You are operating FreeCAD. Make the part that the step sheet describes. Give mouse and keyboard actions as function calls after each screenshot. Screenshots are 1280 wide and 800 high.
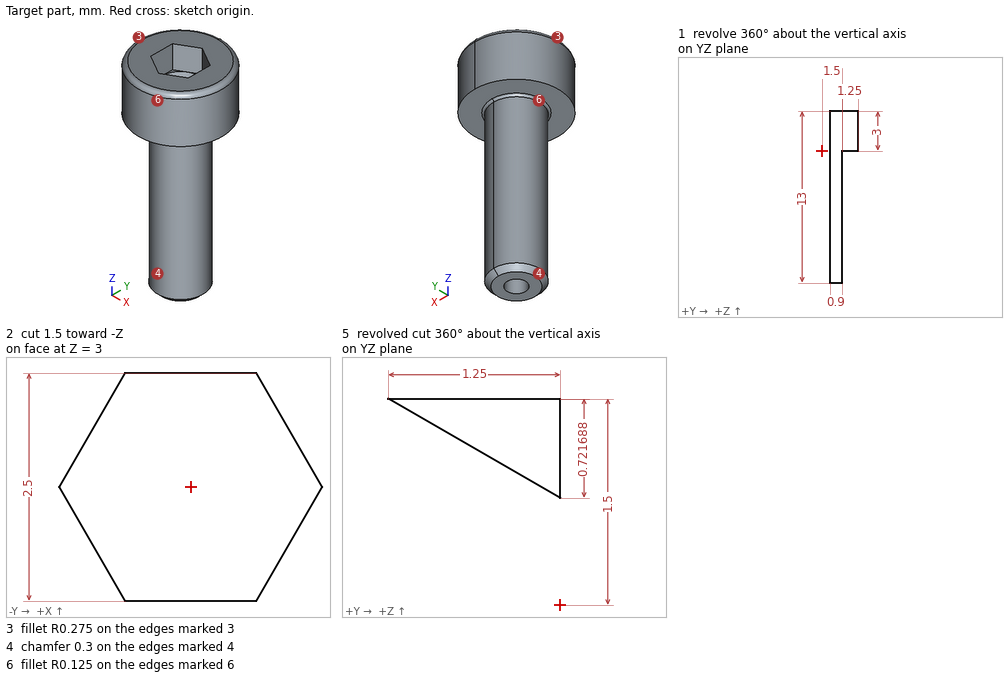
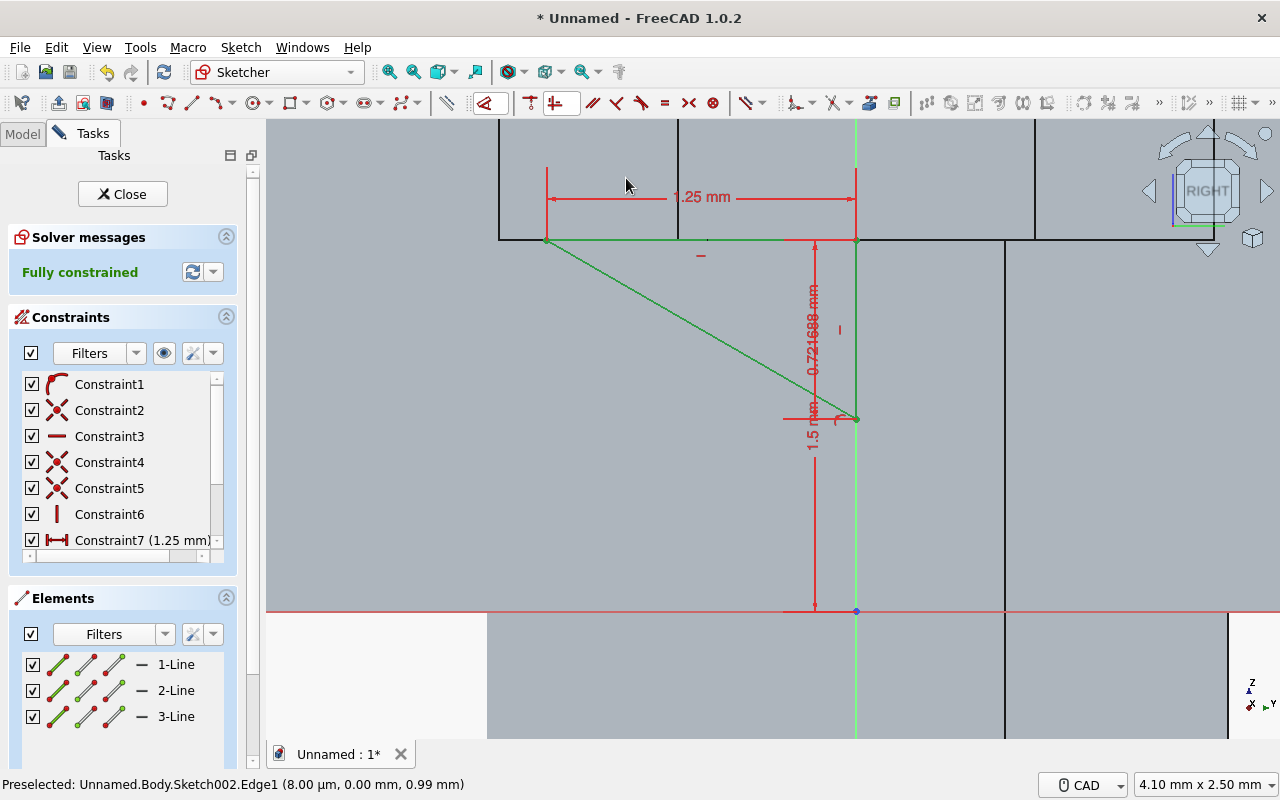
click(123, 194)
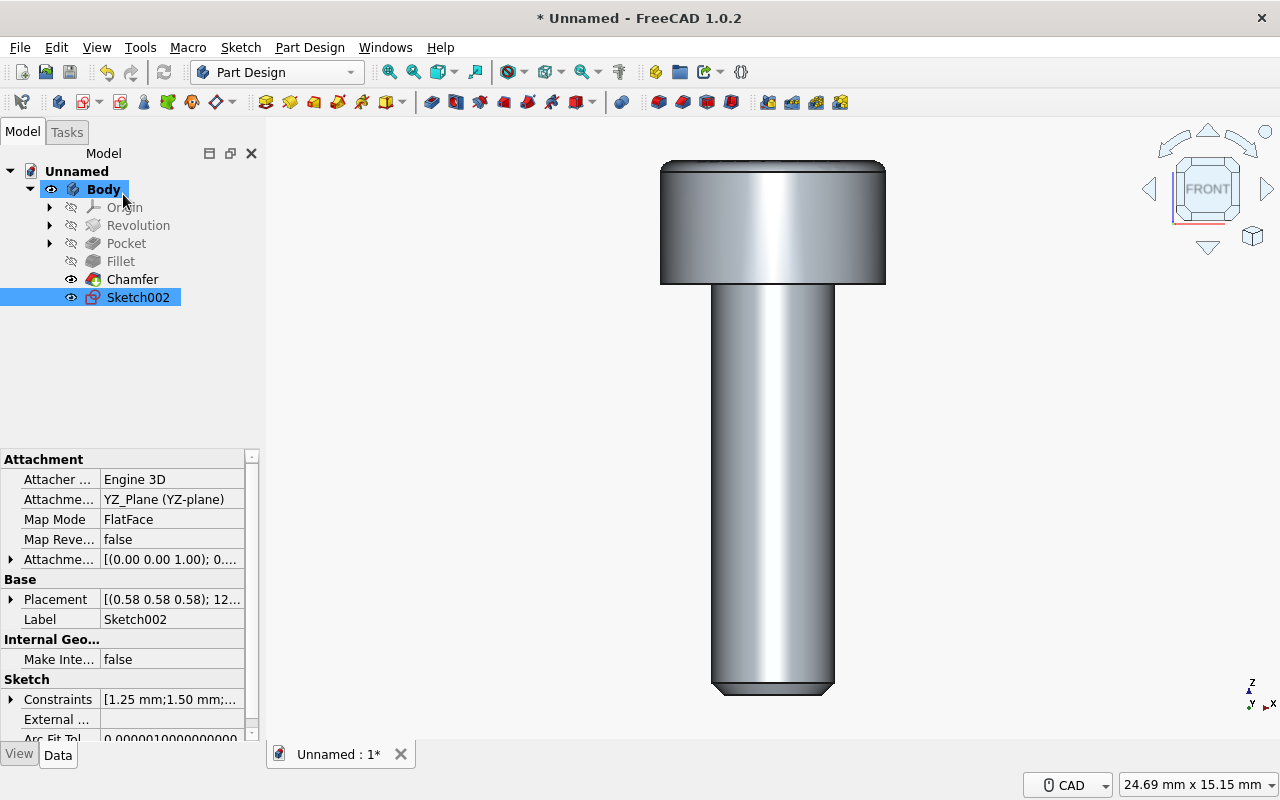
click(480, 102)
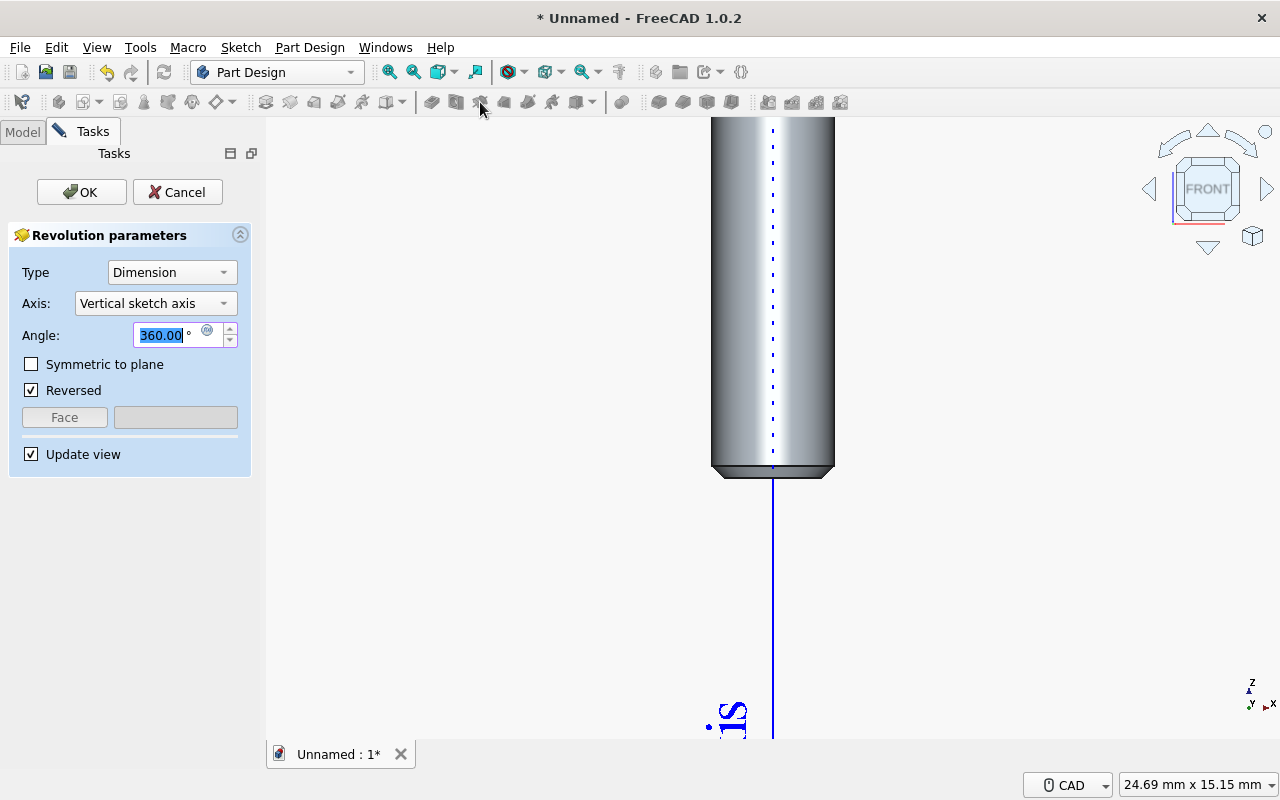
click(82, 192)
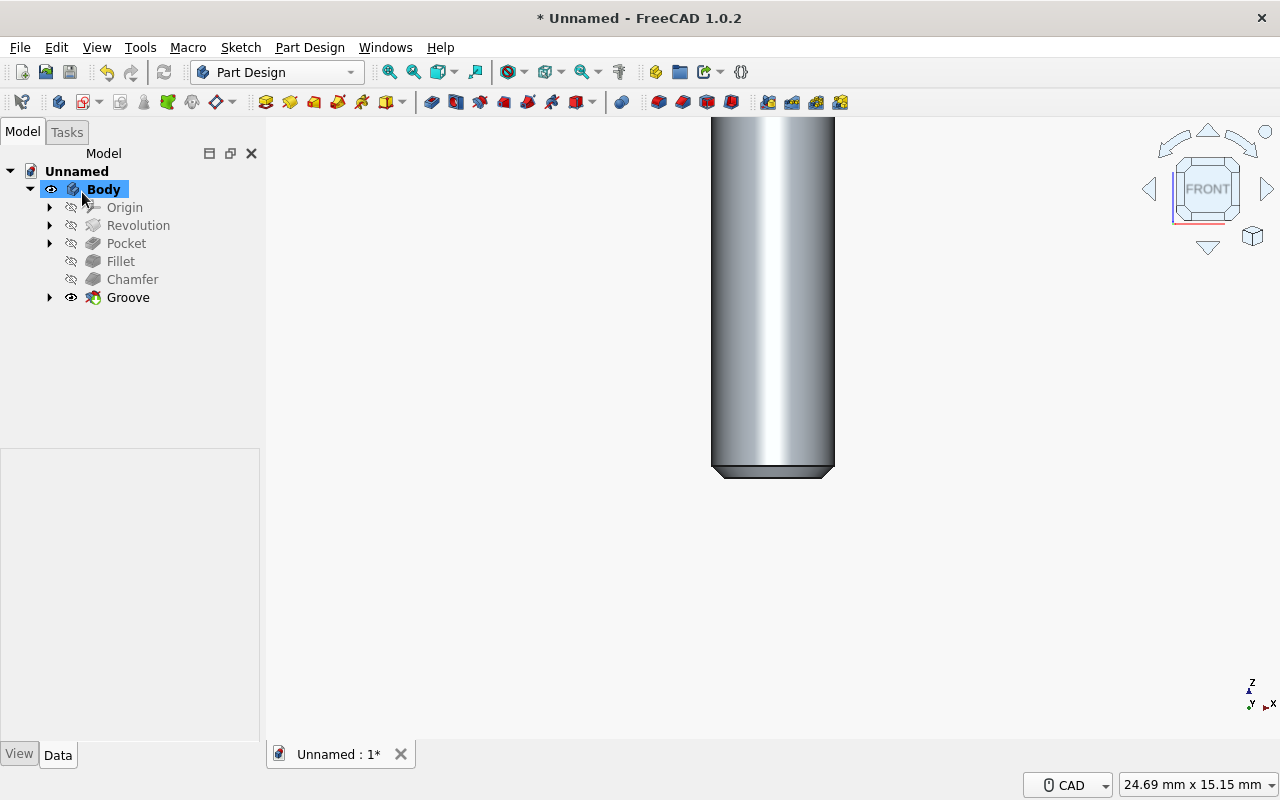
click(390, 72)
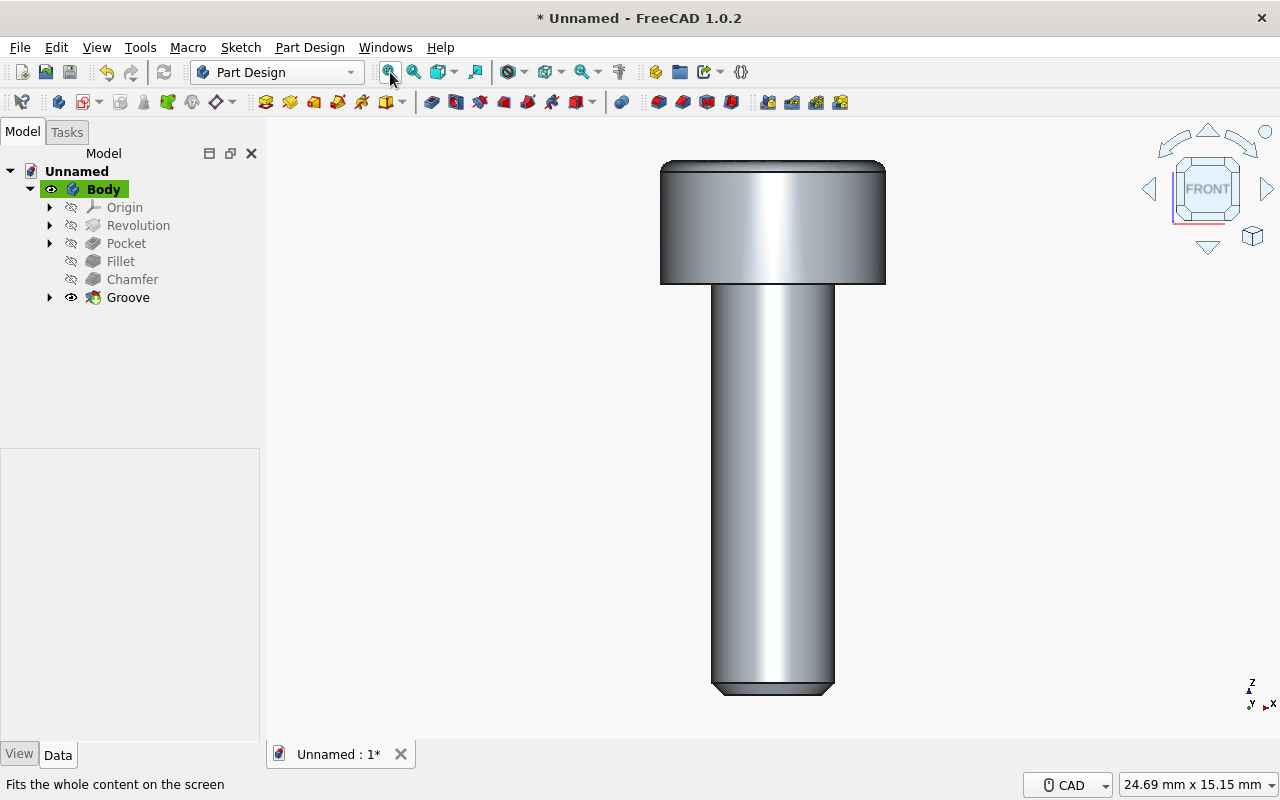
key(0)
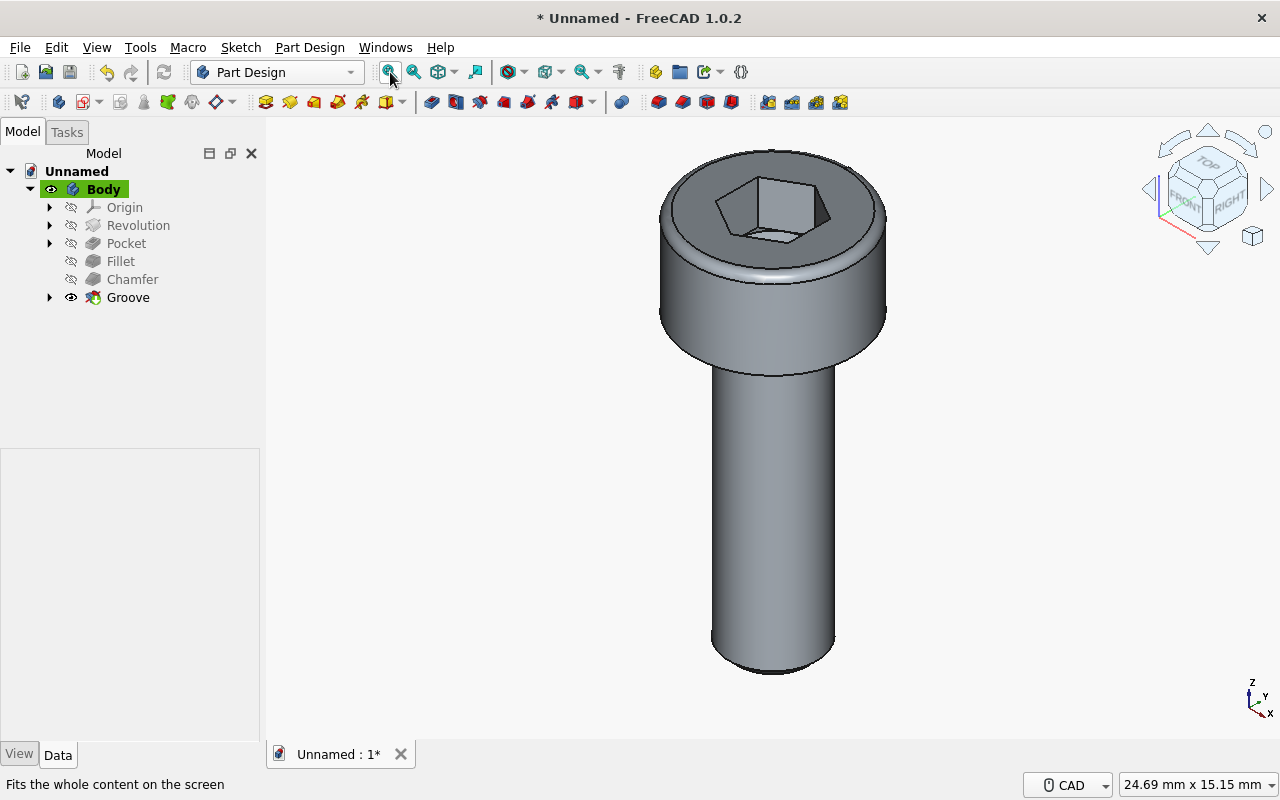
key(2)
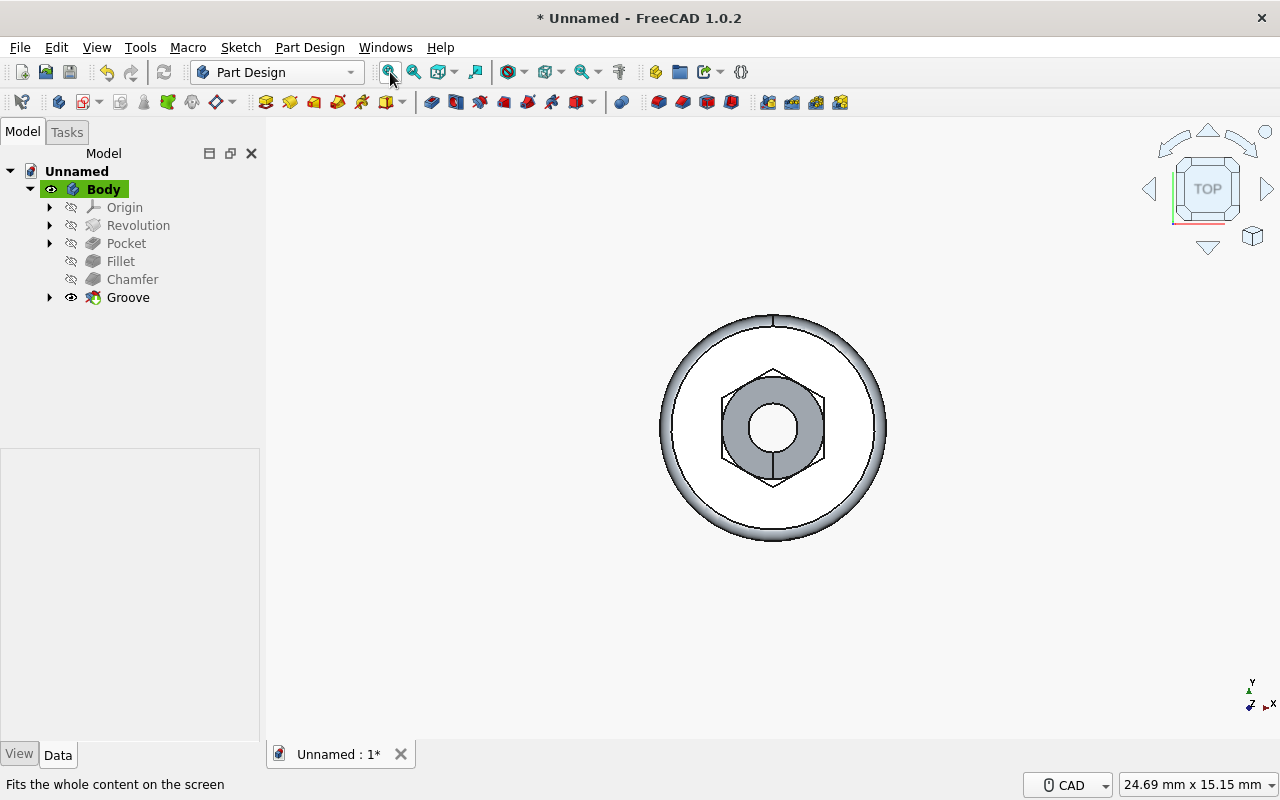
click(390, 72)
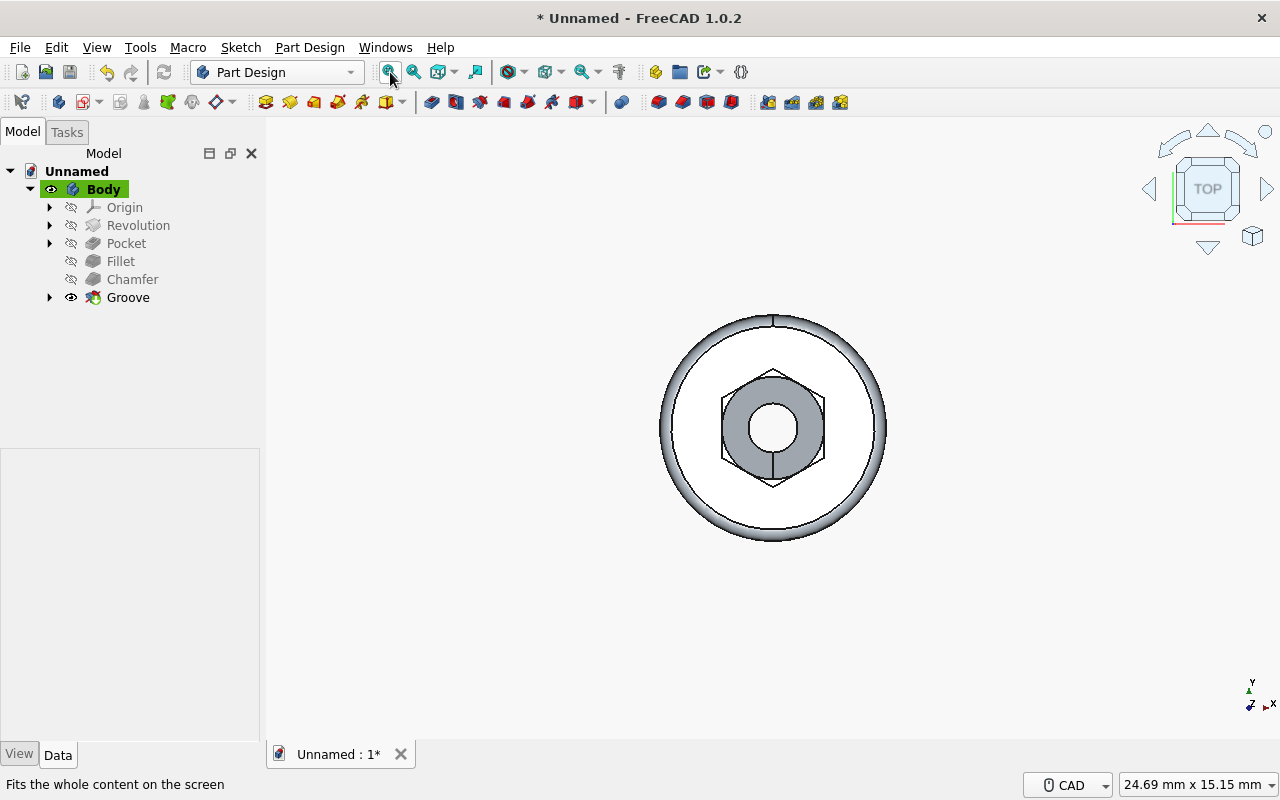
key(1)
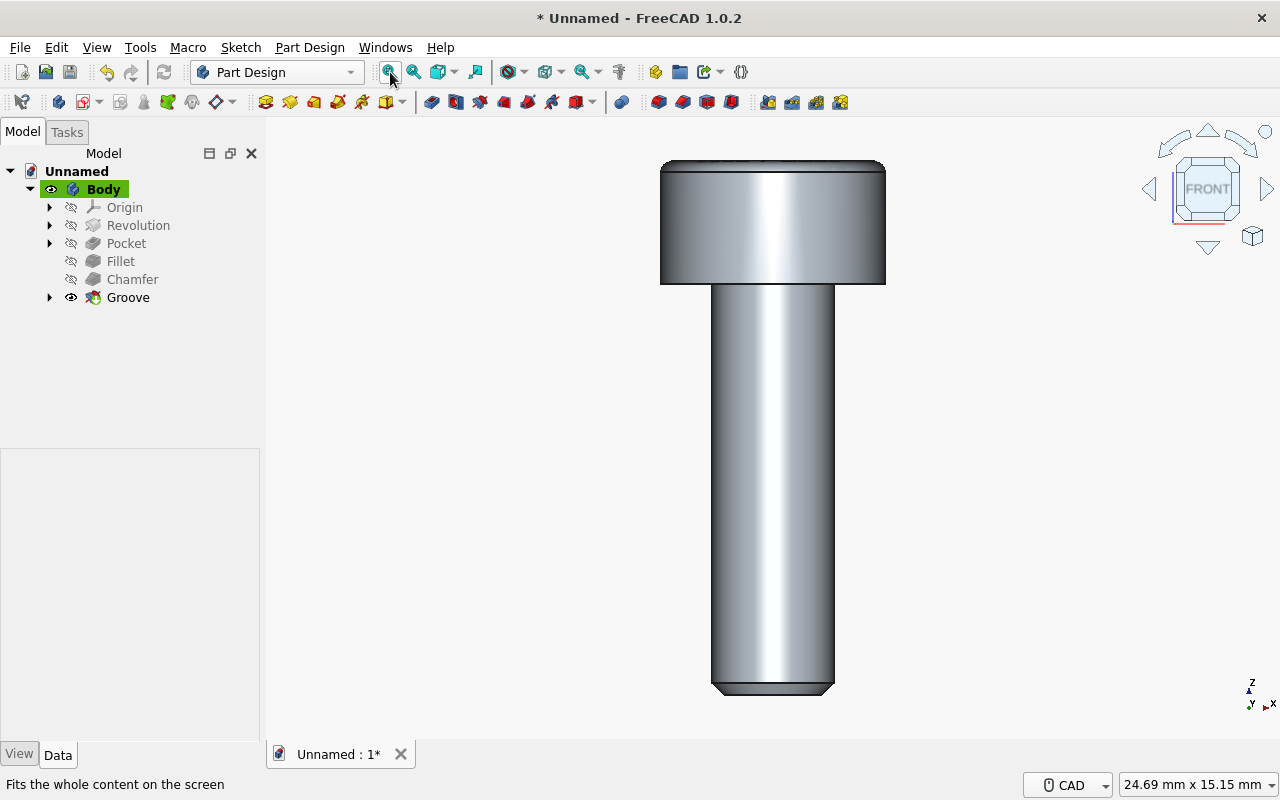
key(3)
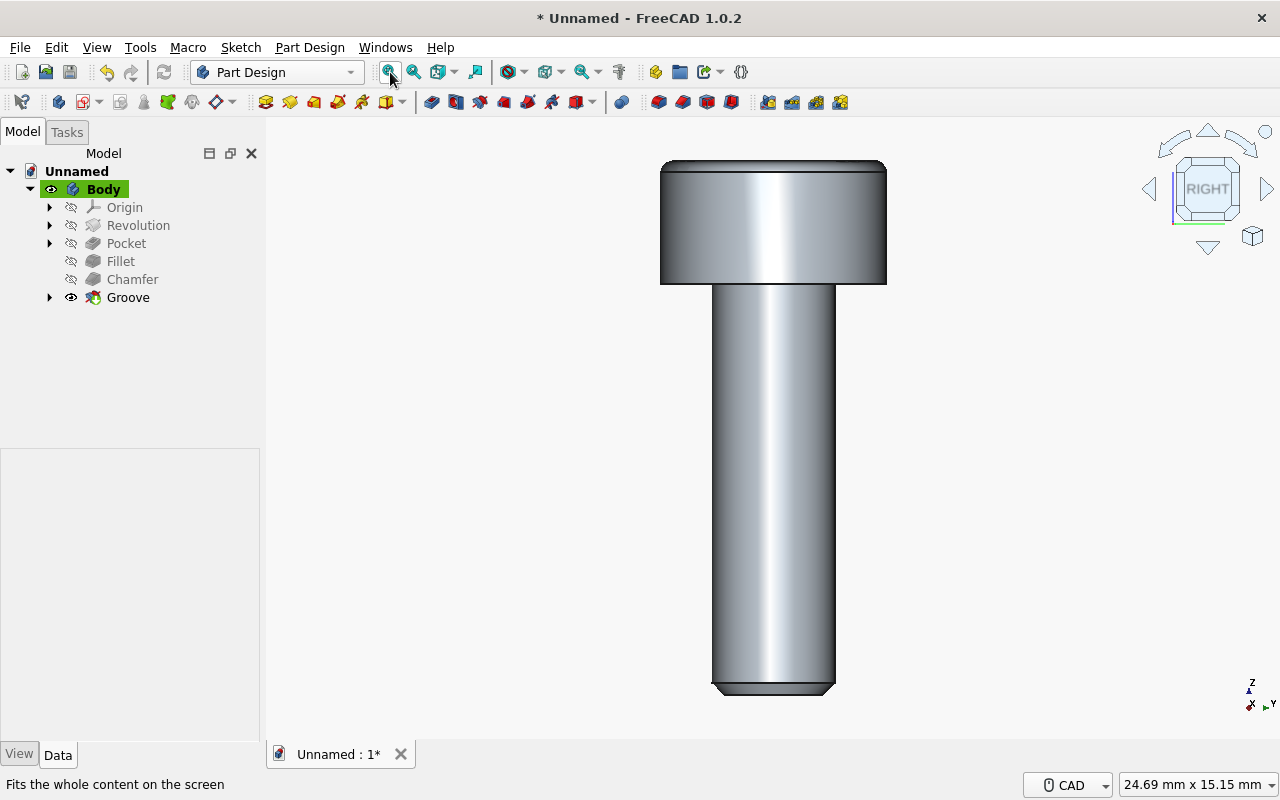
key(5)